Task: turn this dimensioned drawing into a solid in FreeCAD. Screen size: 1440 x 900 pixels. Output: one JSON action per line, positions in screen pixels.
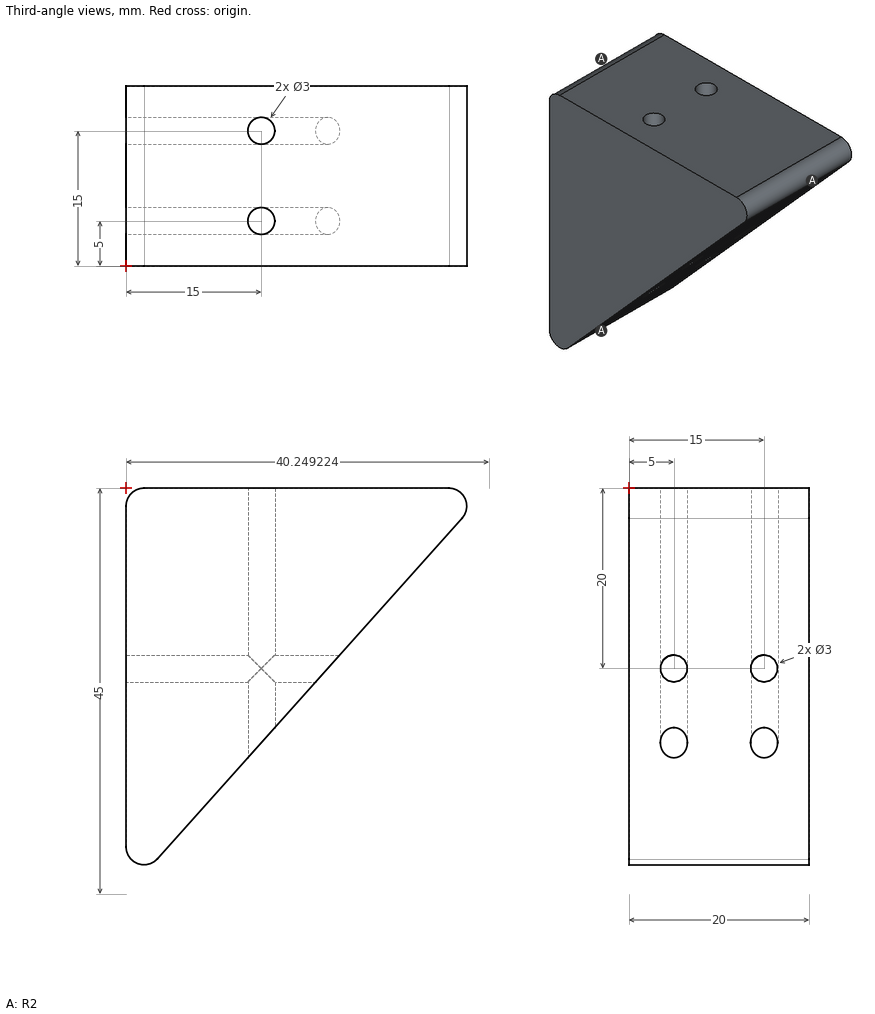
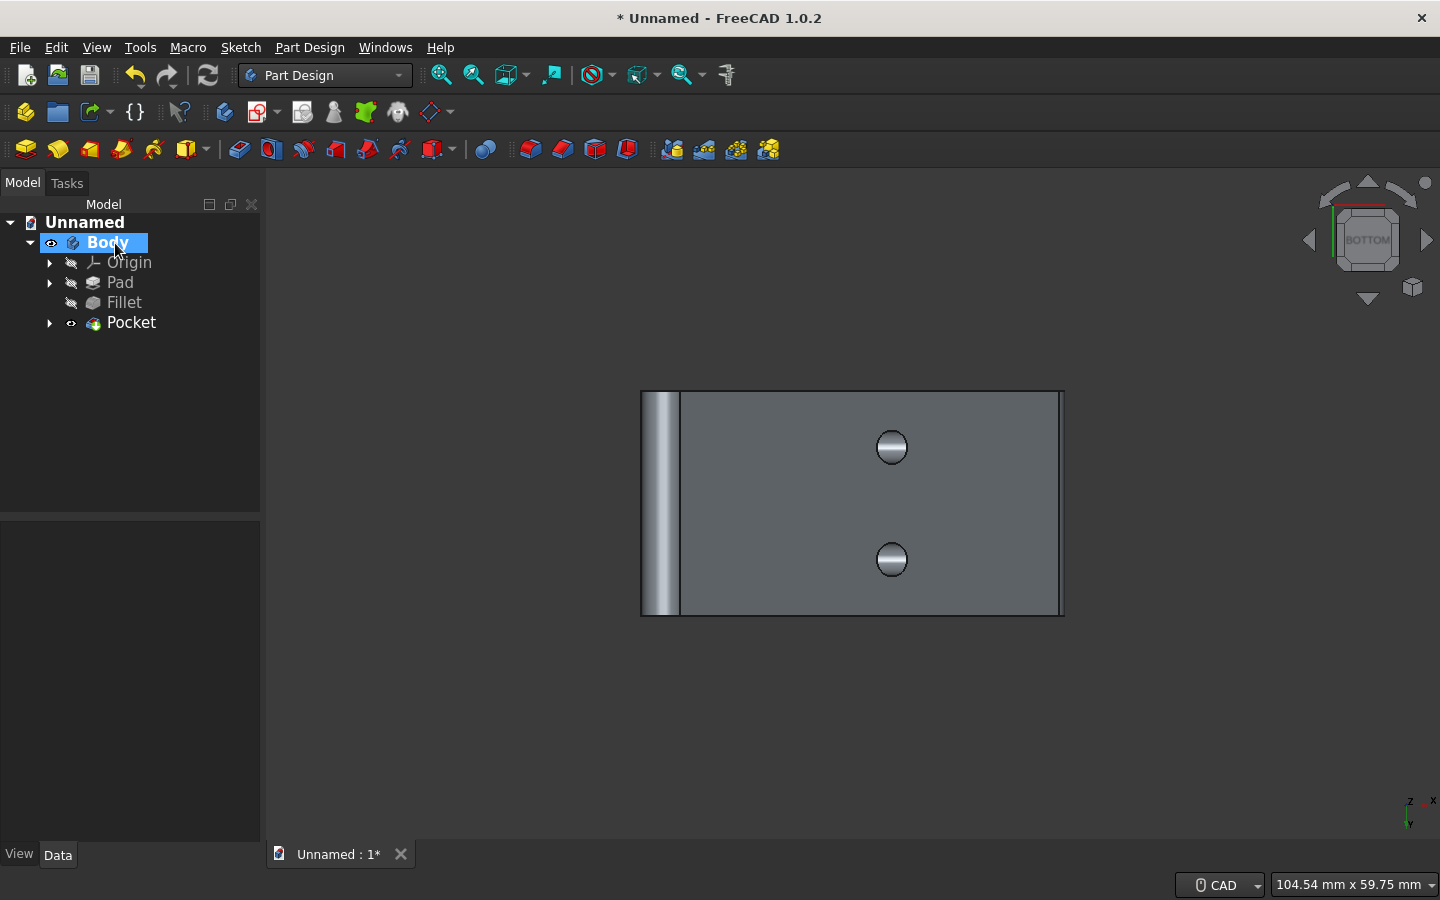
{"action": "left_click", "coordinate": [258, 112]}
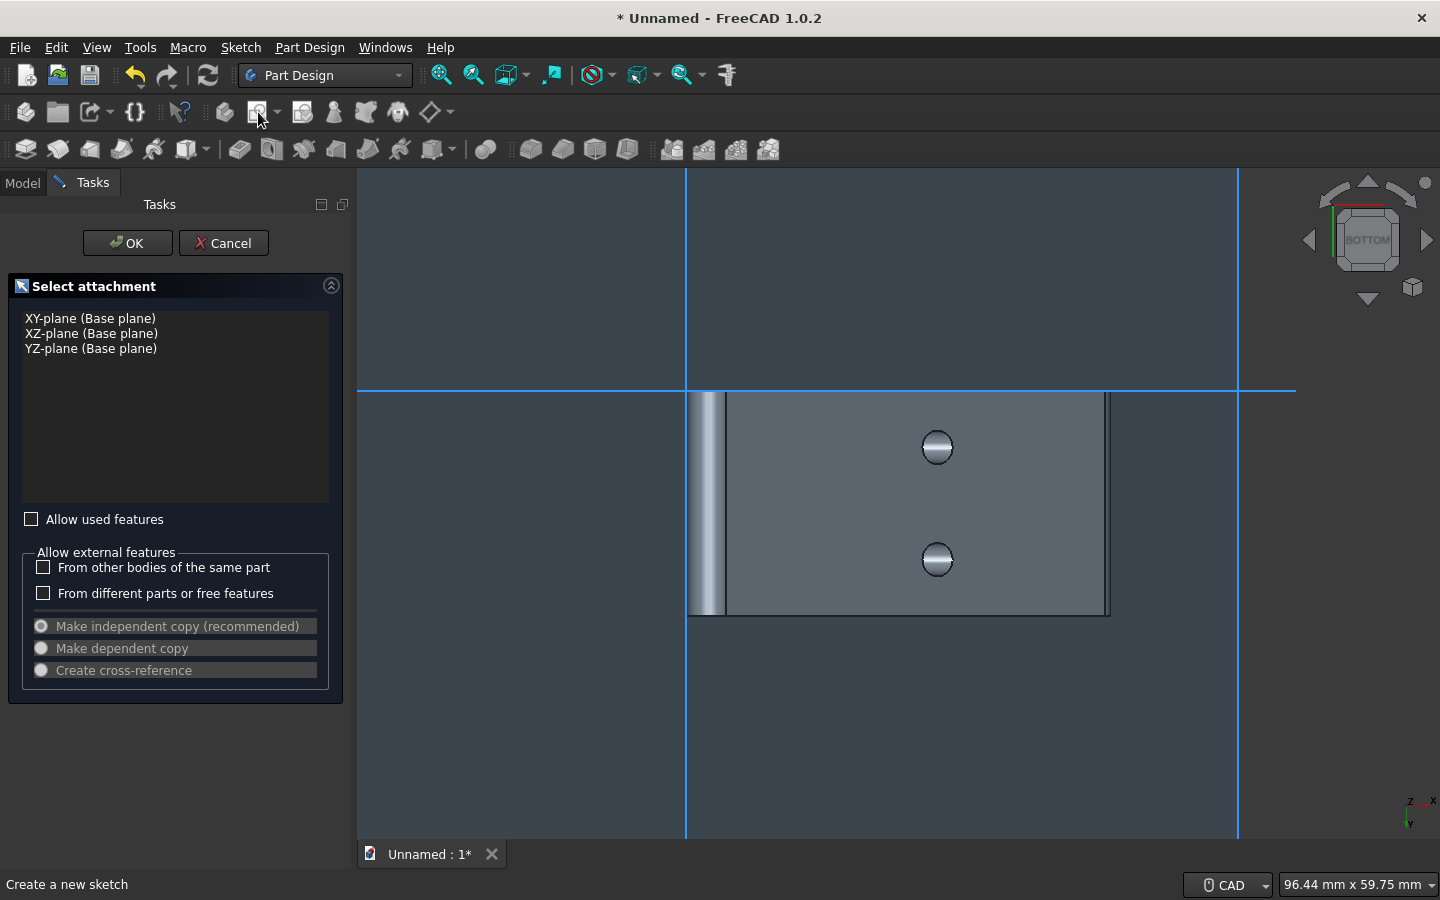
{"action": "left_click", "coordinate": [82, 318]}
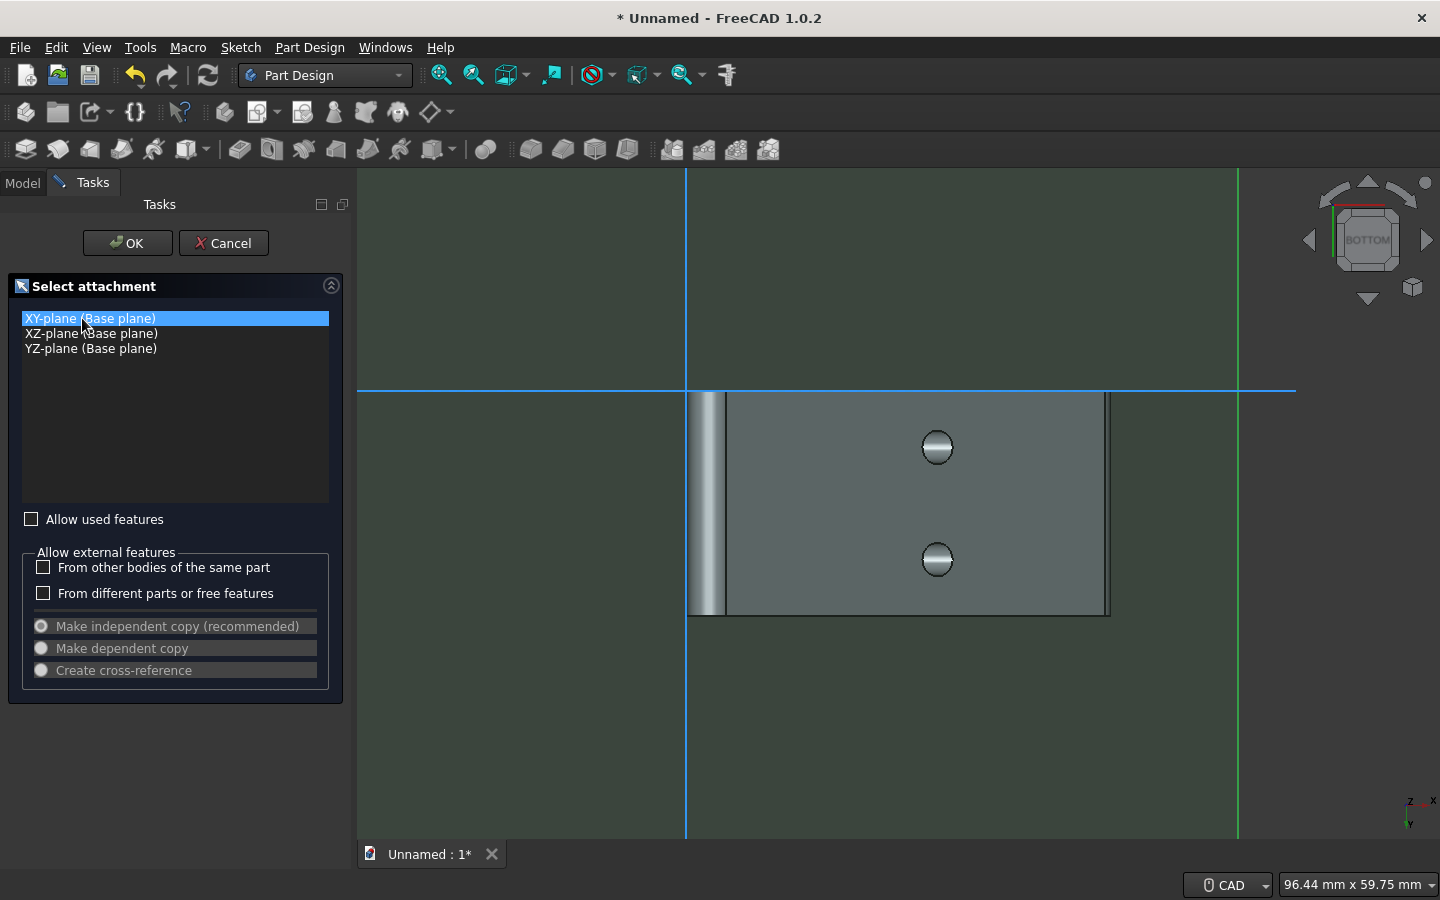
{"action": "left_click", "coordinate": [128, 243]}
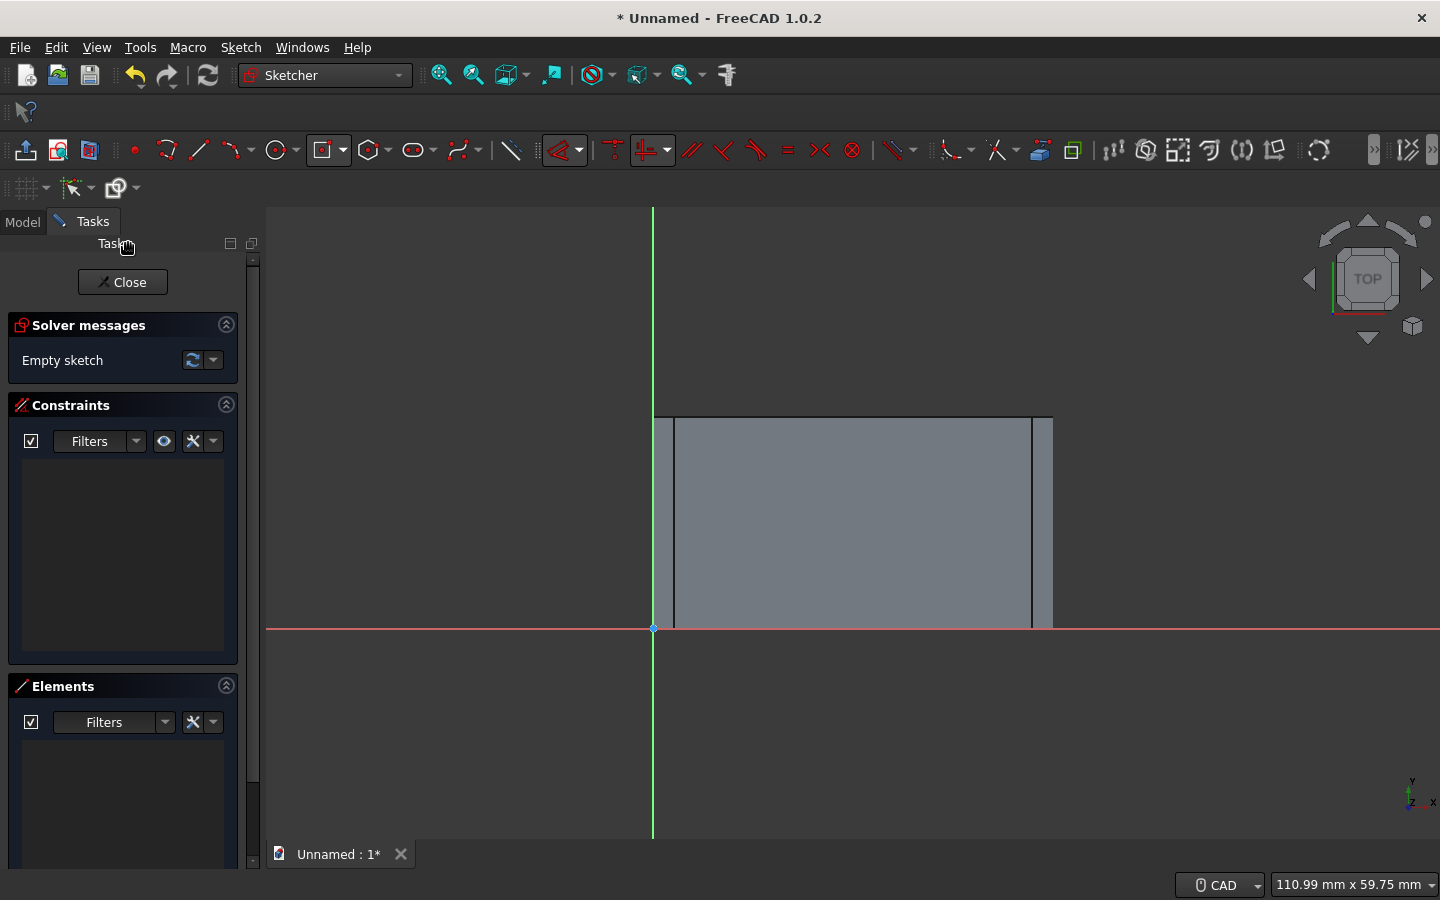
{"action": "scroll", "coordinate": [705, 557], "scroll_direction": "up", "scroll_amount": 4}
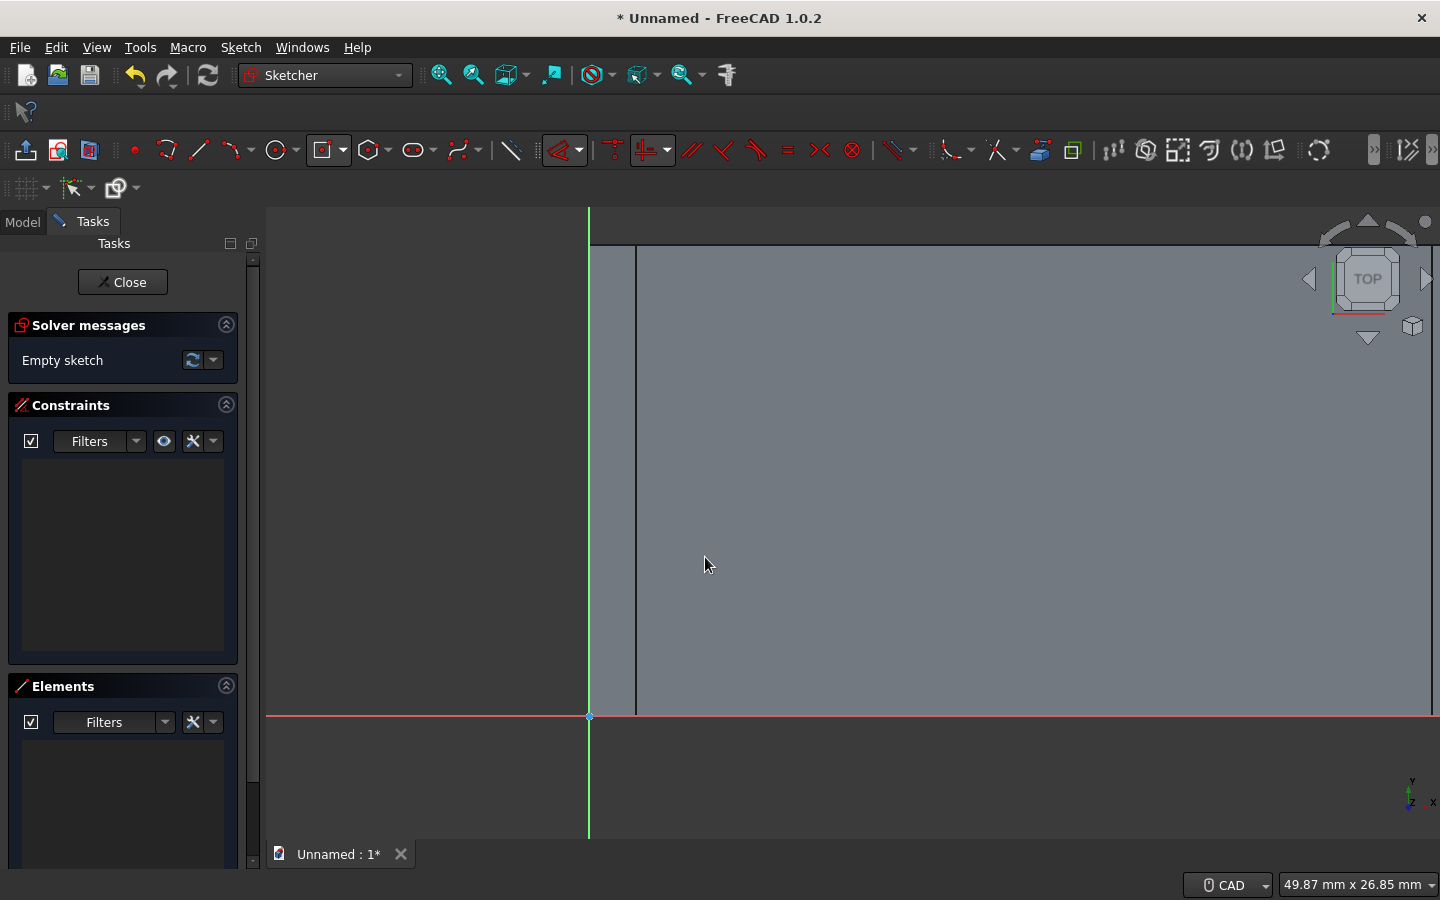
{"action": "left_click", "coordinate": [276, 150]}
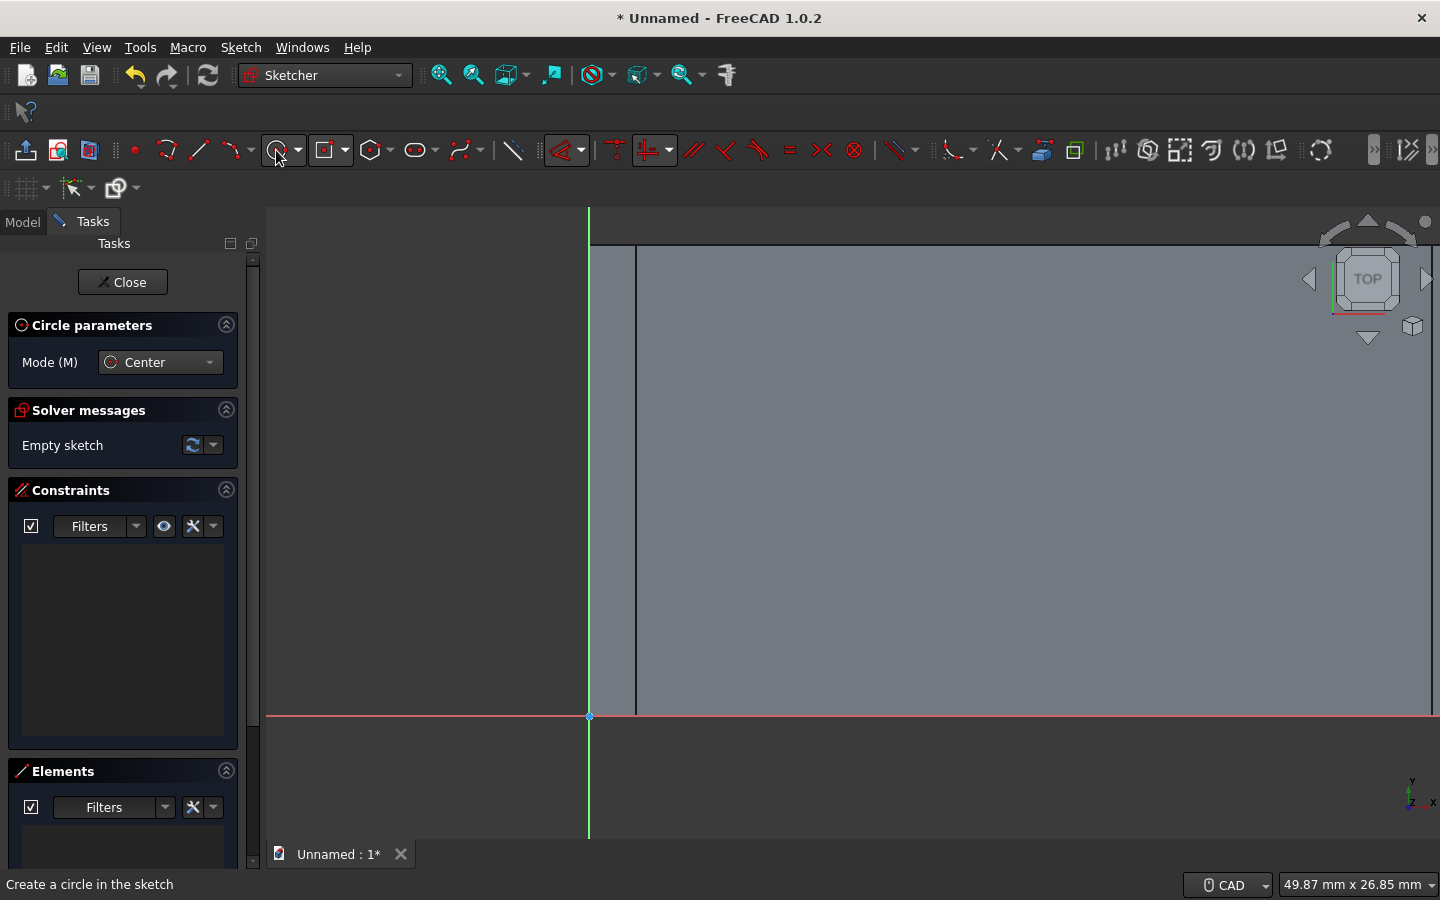
{"action": "left_click", "coordinate": [942, 363]}
{"action": "mouse_move", "coordinate": [967, 338]}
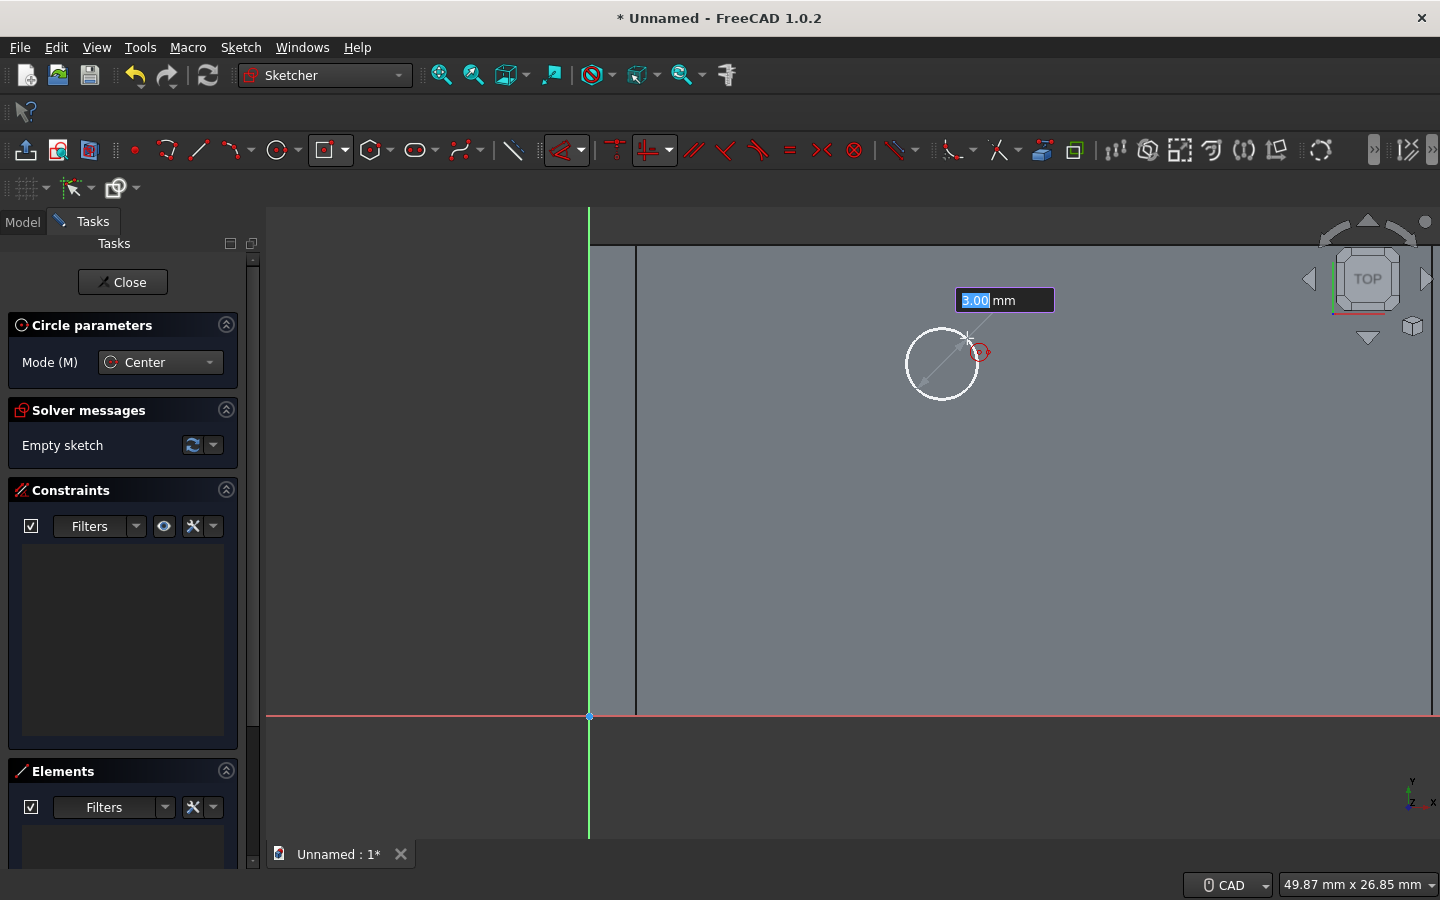
{"action": "type", "text": "3"}
{"action": "key", "text": "Return"}